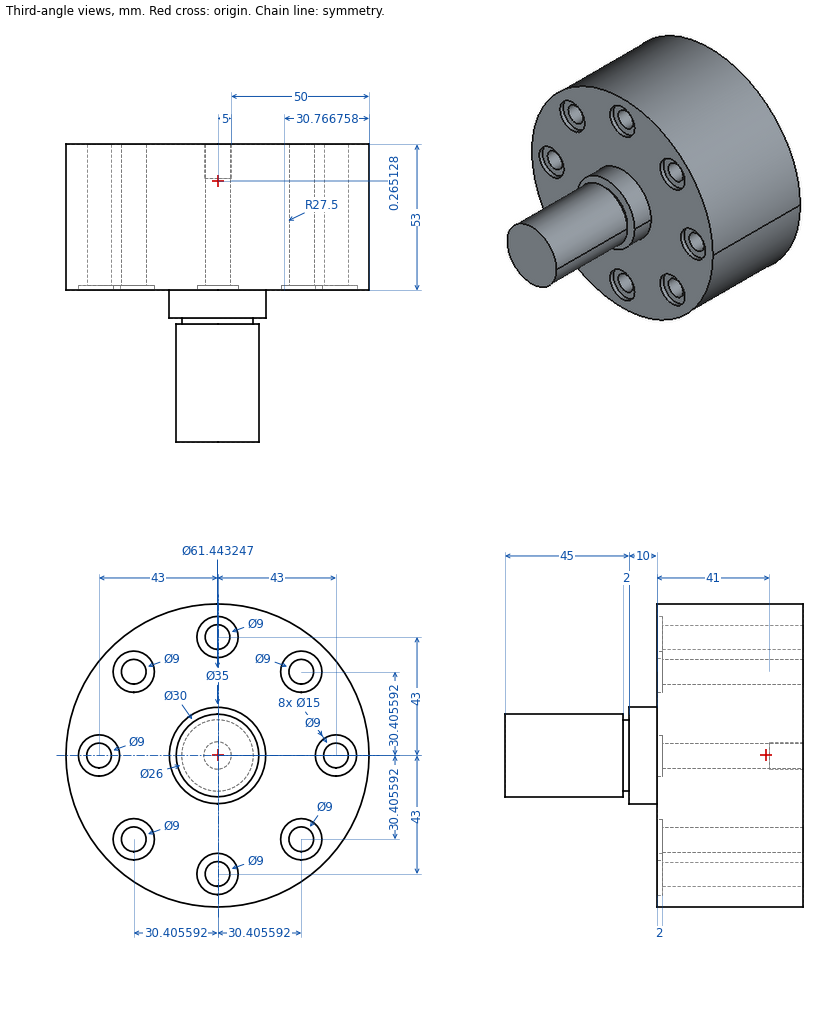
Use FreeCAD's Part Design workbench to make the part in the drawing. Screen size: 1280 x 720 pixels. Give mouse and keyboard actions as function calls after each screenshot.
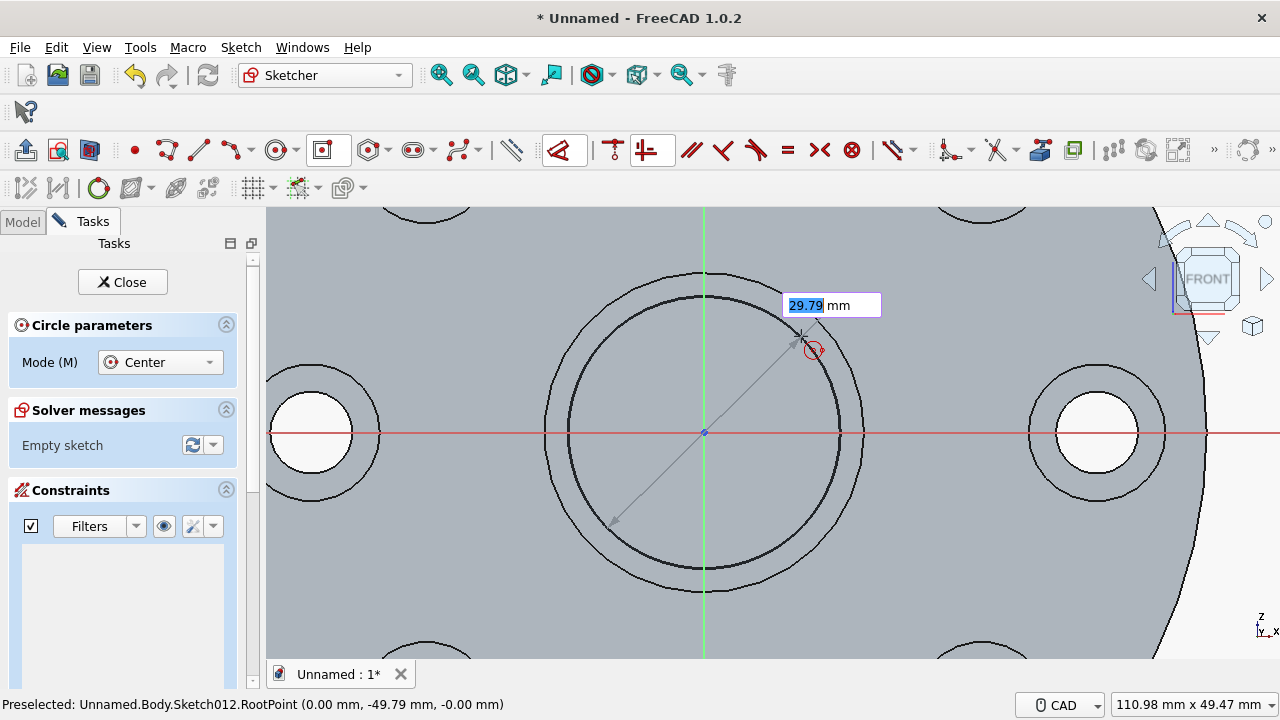
text(30)
key(Return)
key(Escape)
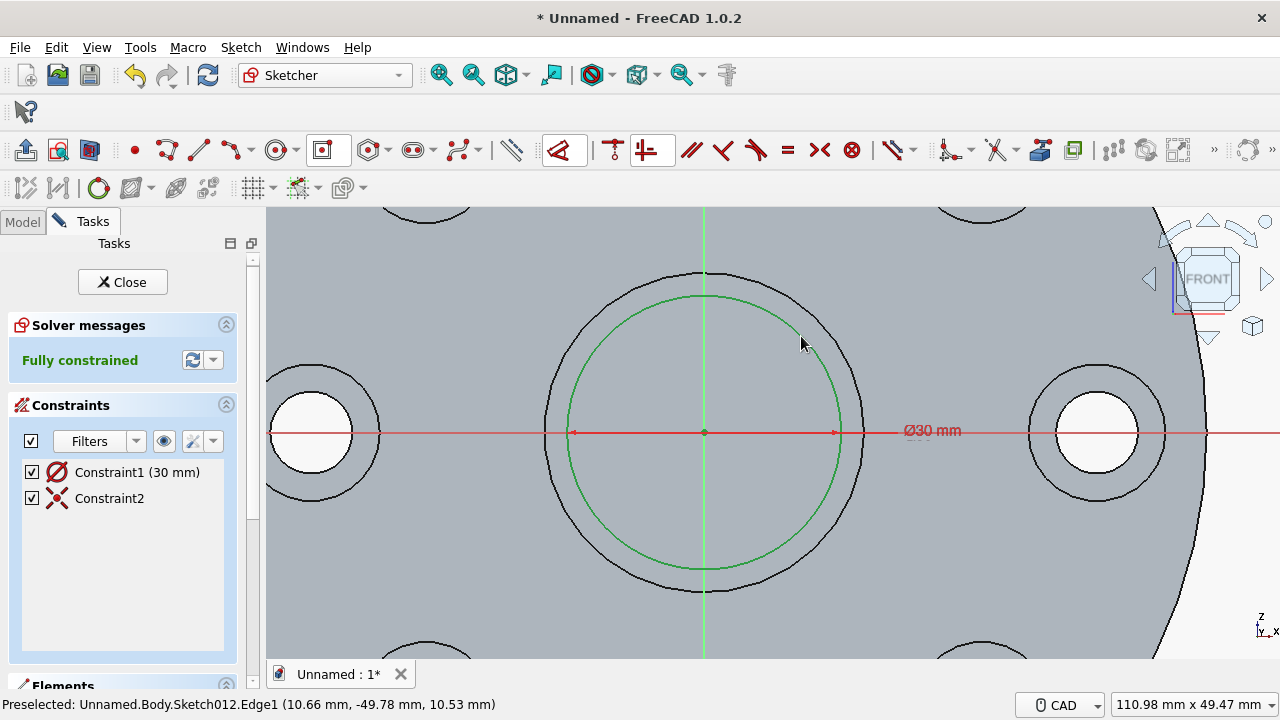
click(123, 282)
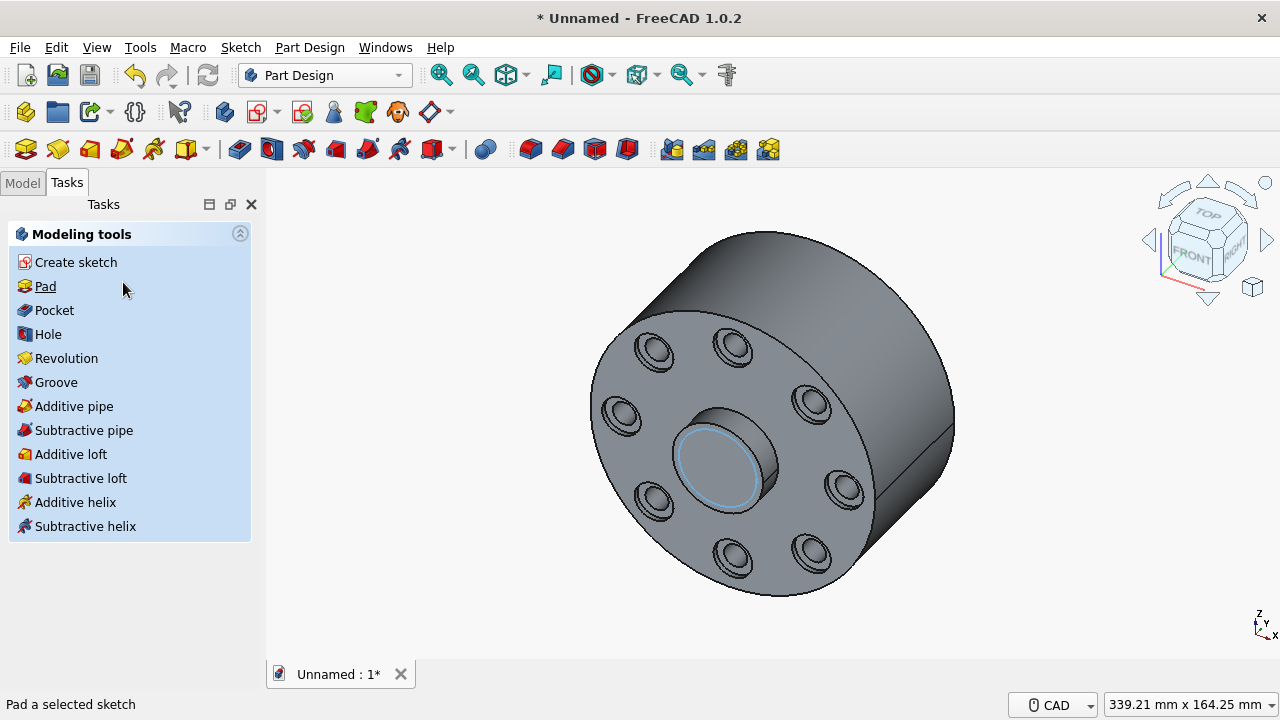
click(26, 150)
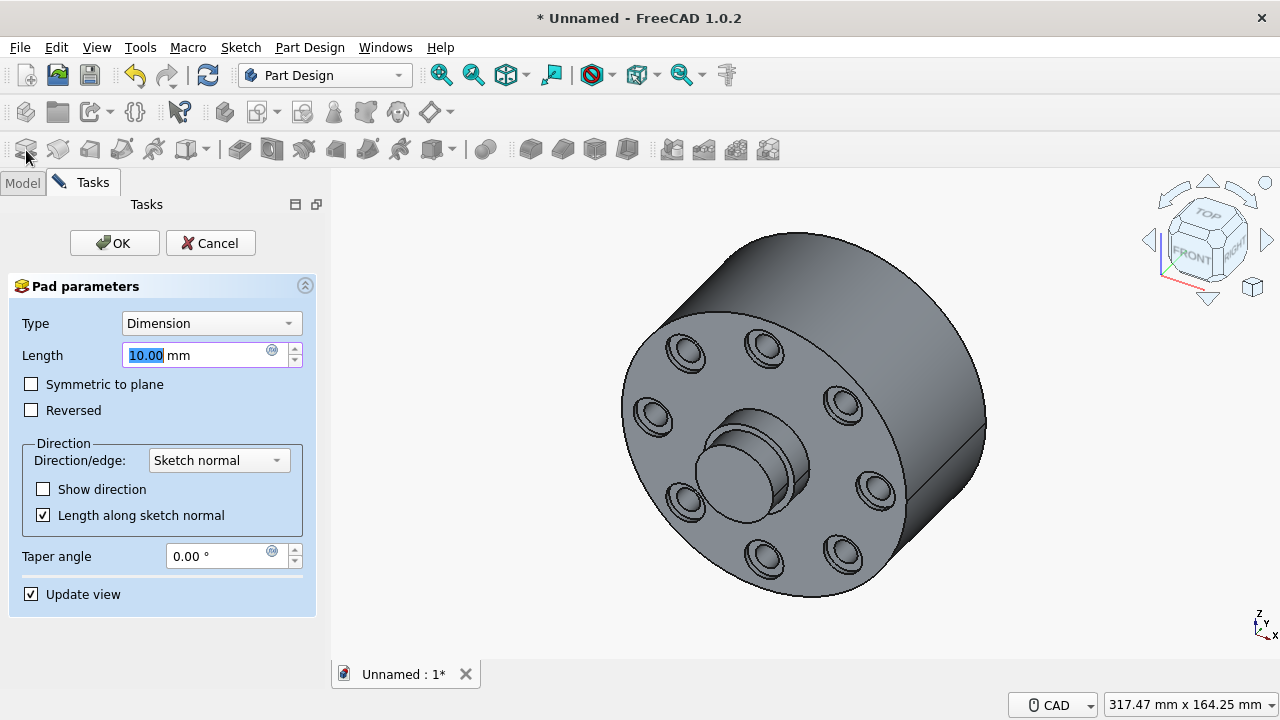
text(45)
key(Tab)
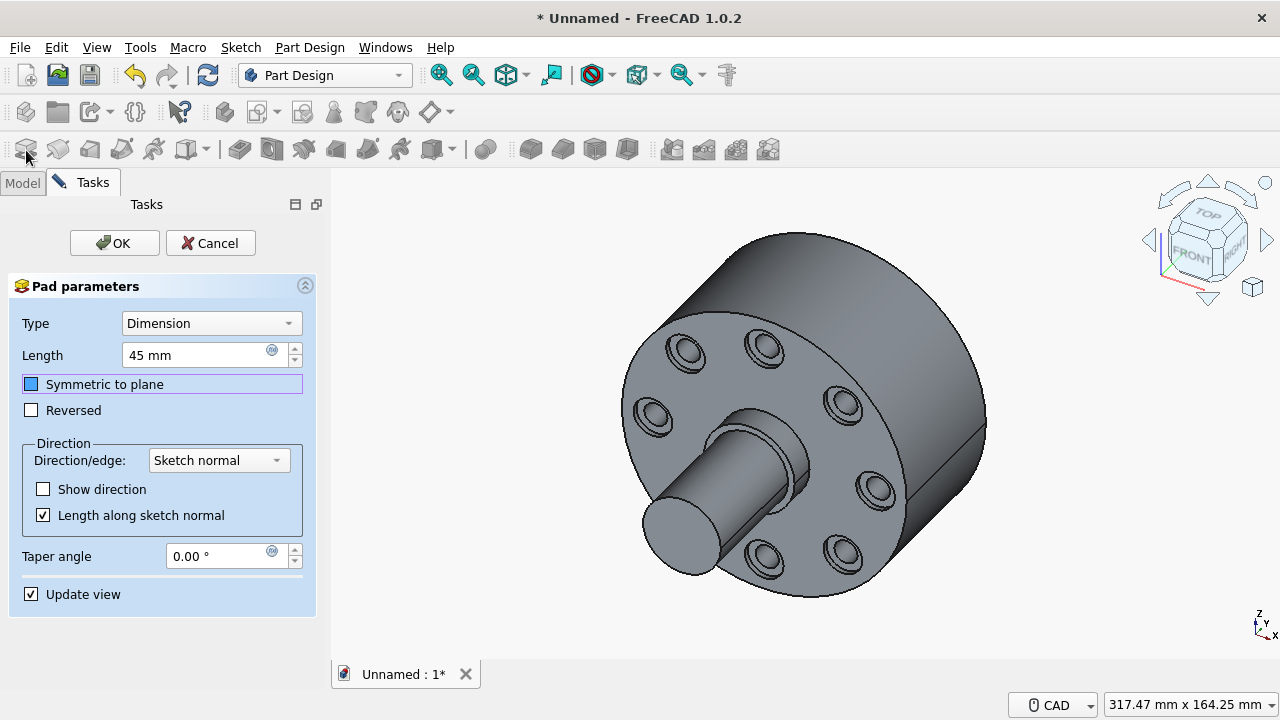
click(115, 243)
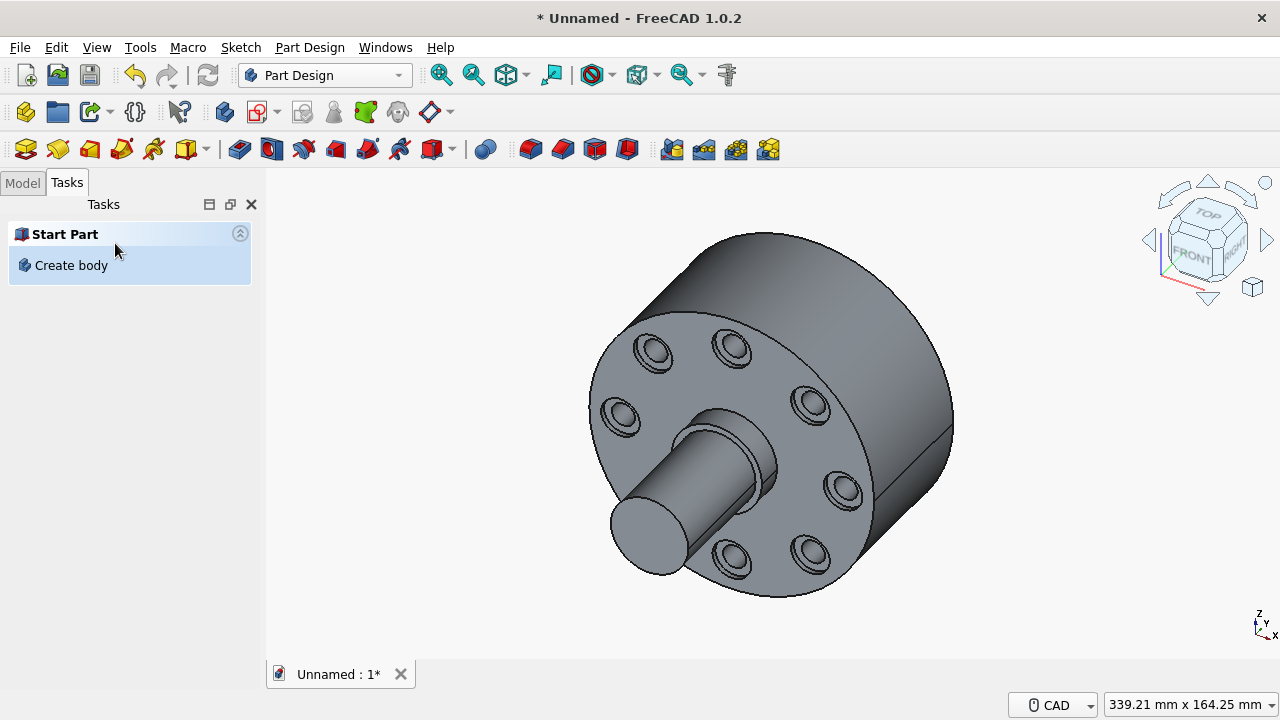
key(v)
key(f)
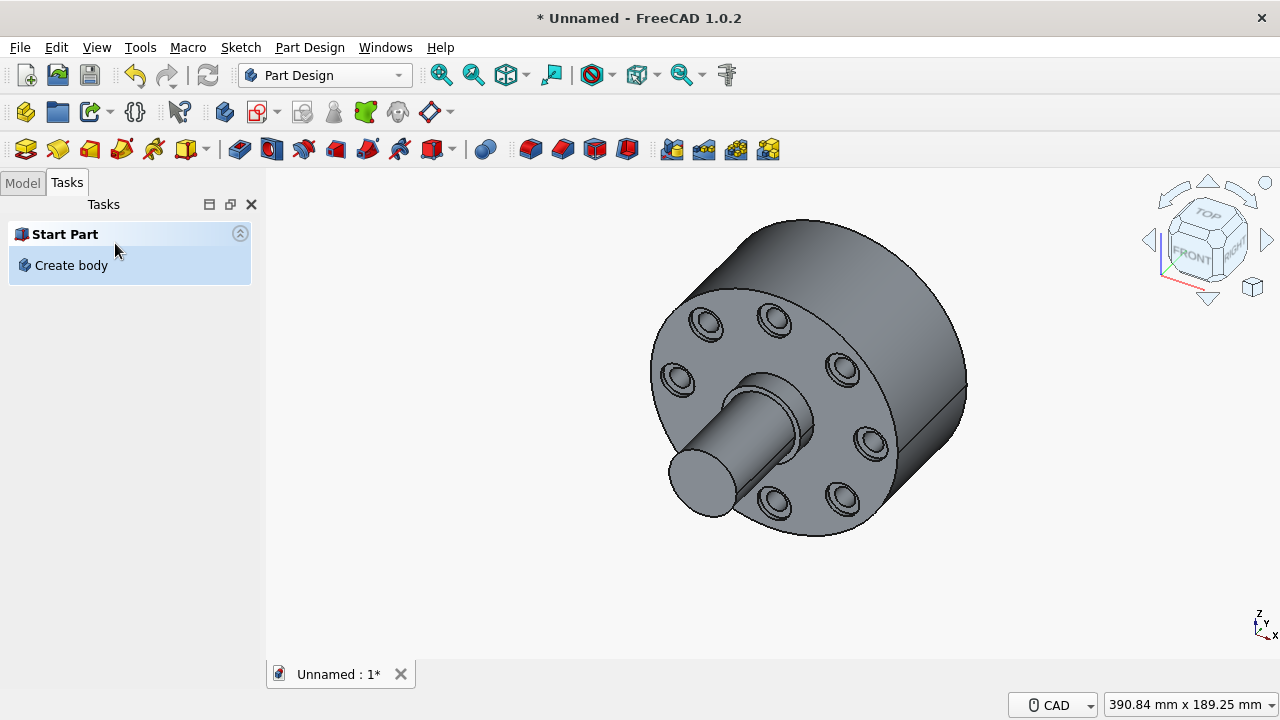
scroll(773, 396, up, 9)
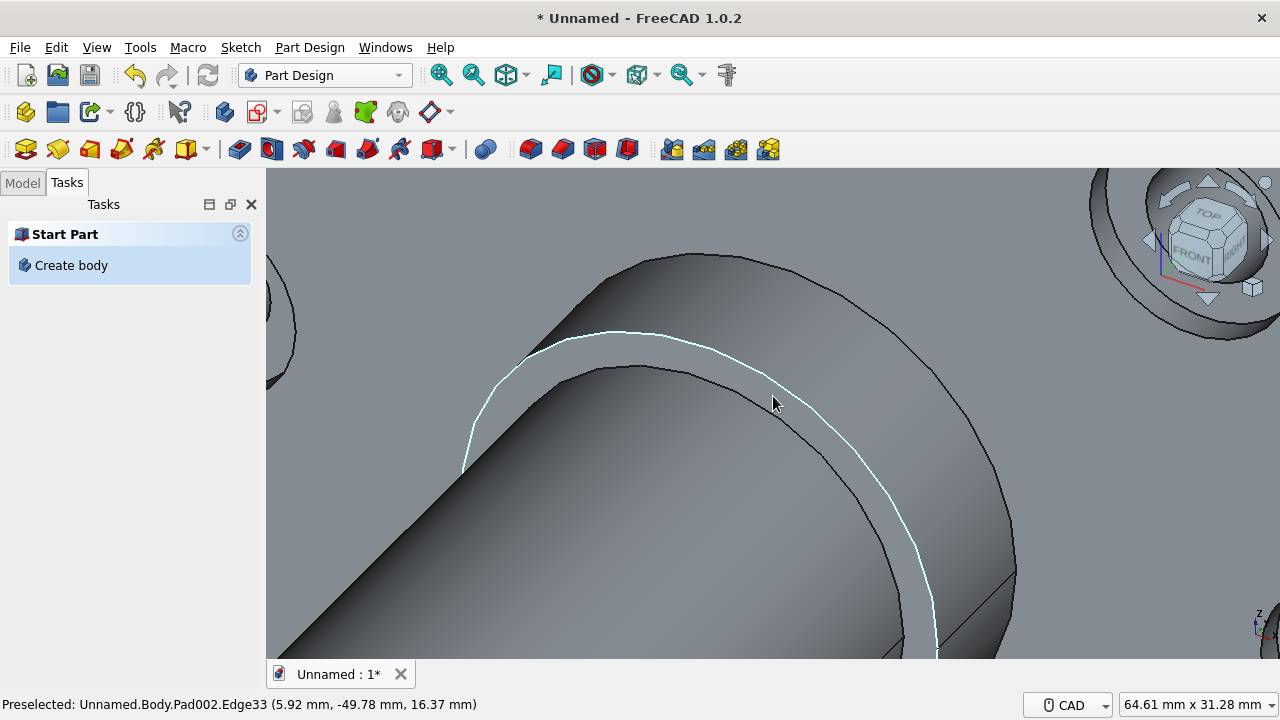
click(768, 398)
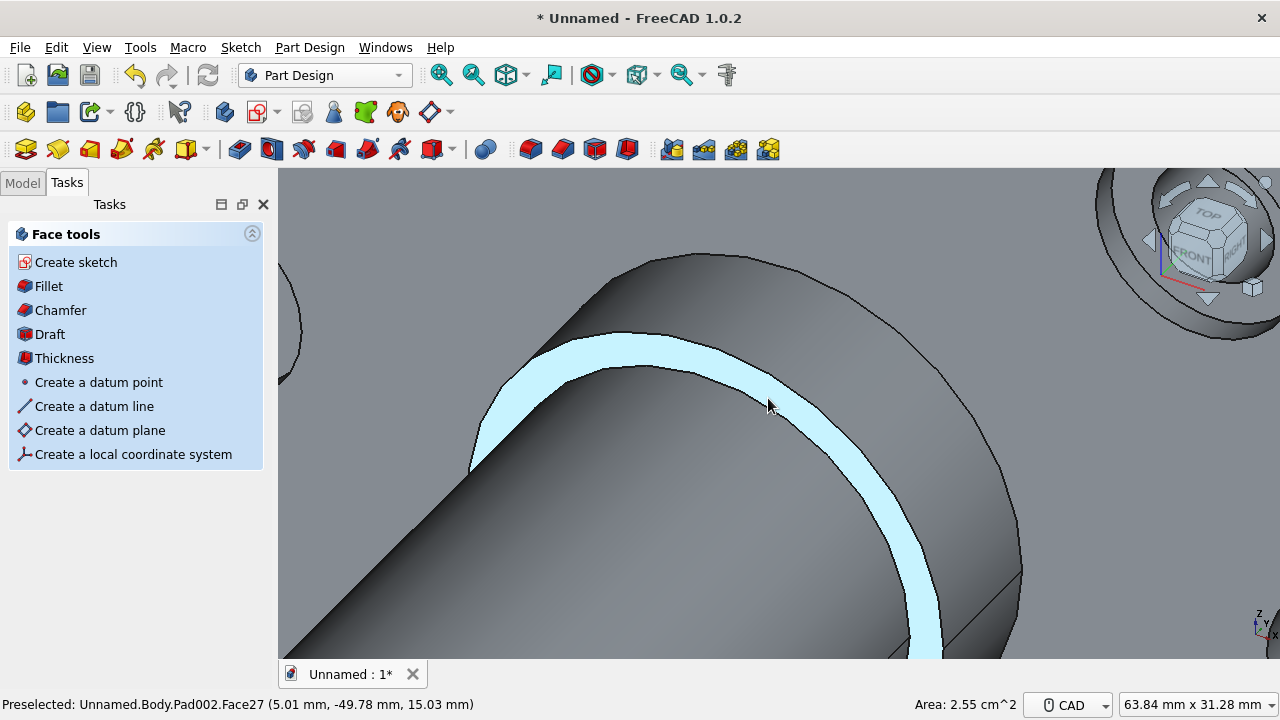
click(258, 112)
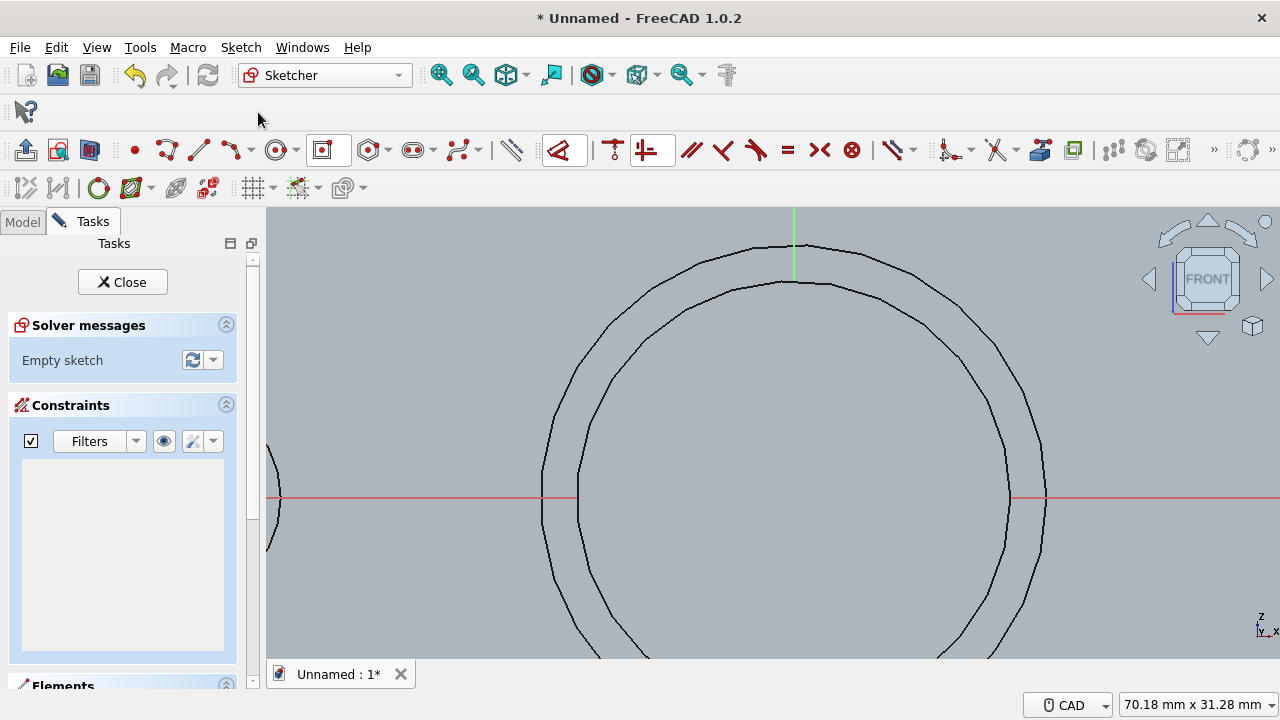
click(90, 150)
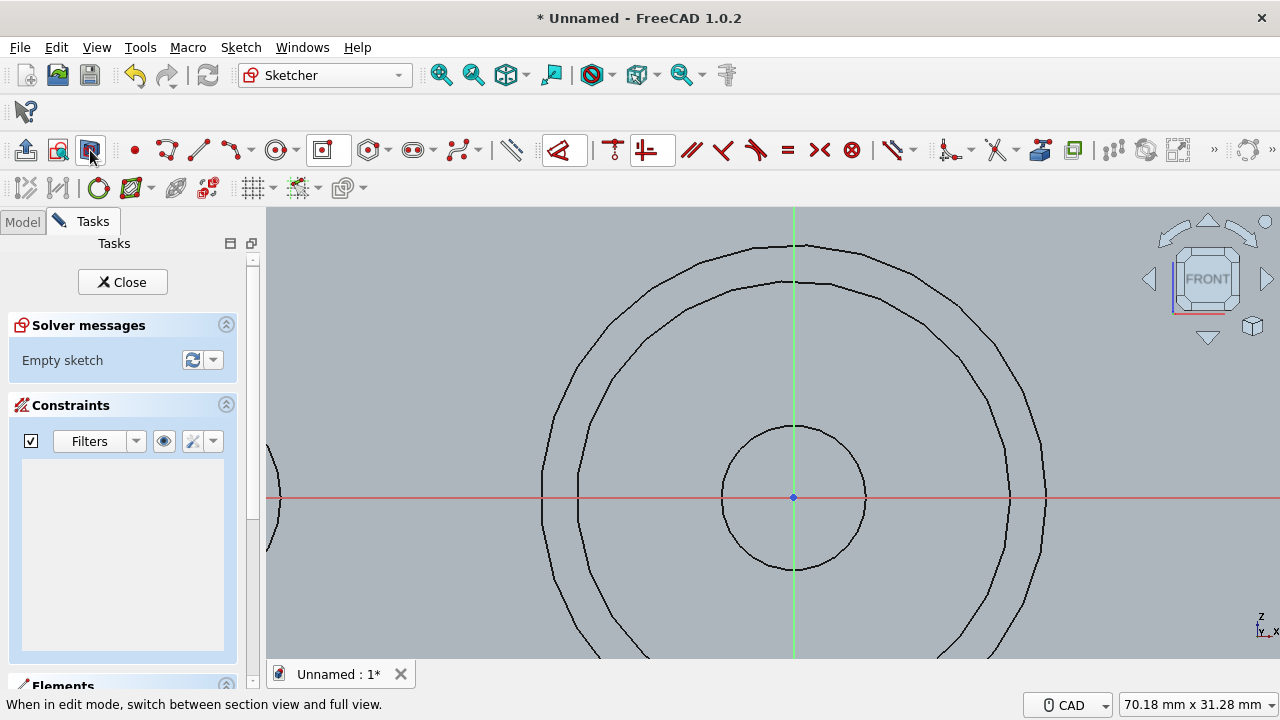
scroll(523, 301, down, 2)